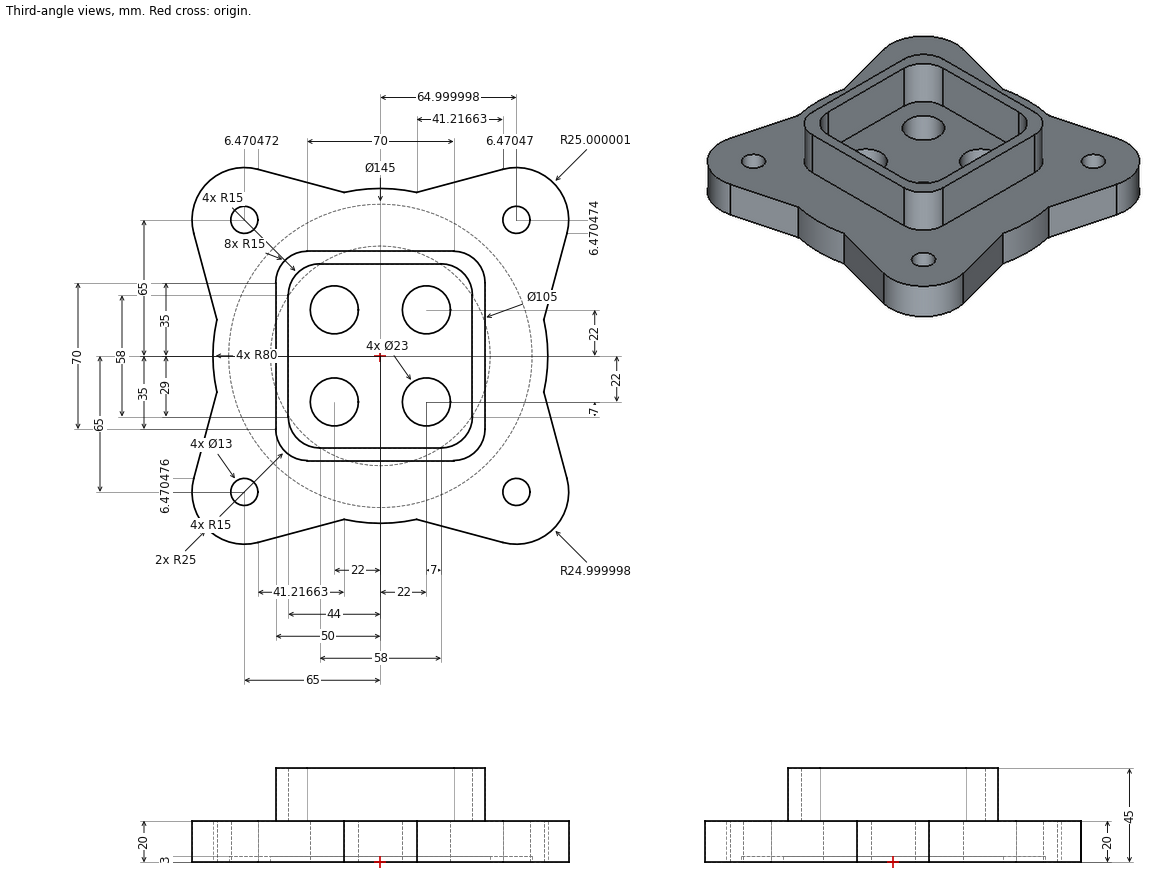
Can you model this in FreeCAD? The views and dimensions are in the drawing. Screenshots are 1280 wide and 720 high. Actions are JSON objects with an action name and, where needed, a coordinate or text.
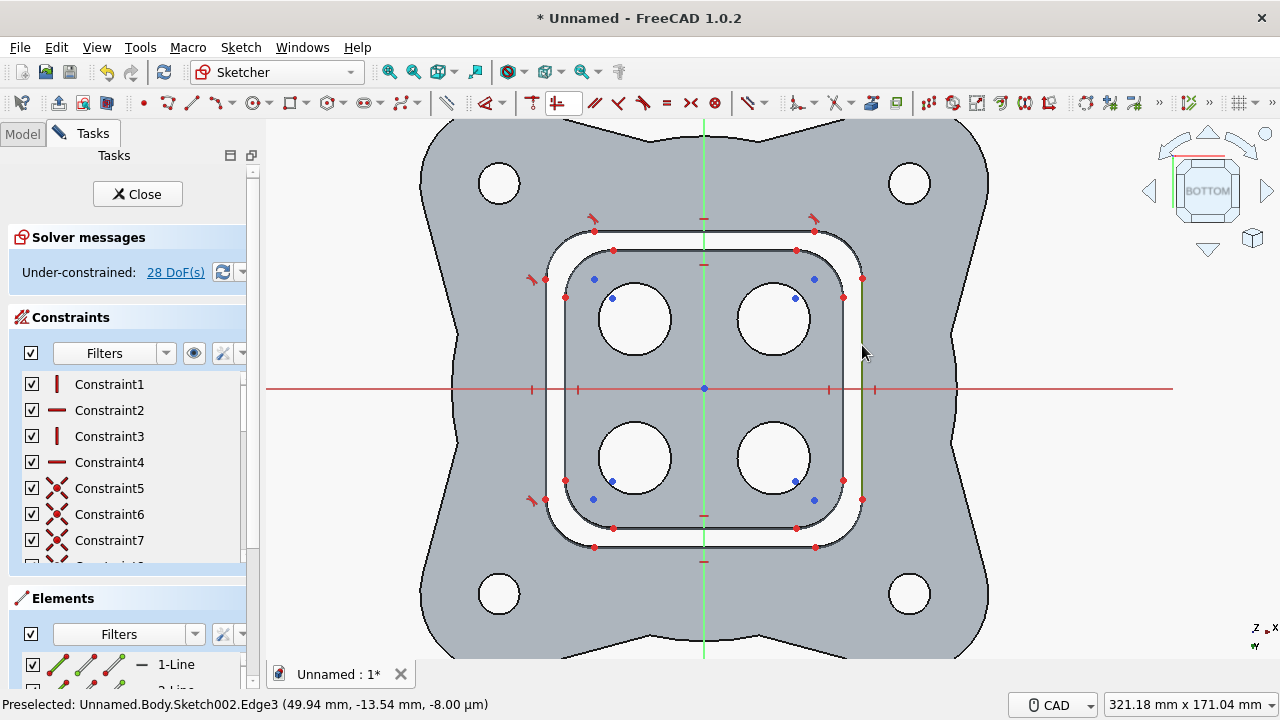
{"action": "left_click", "coordinate": [857, 258]}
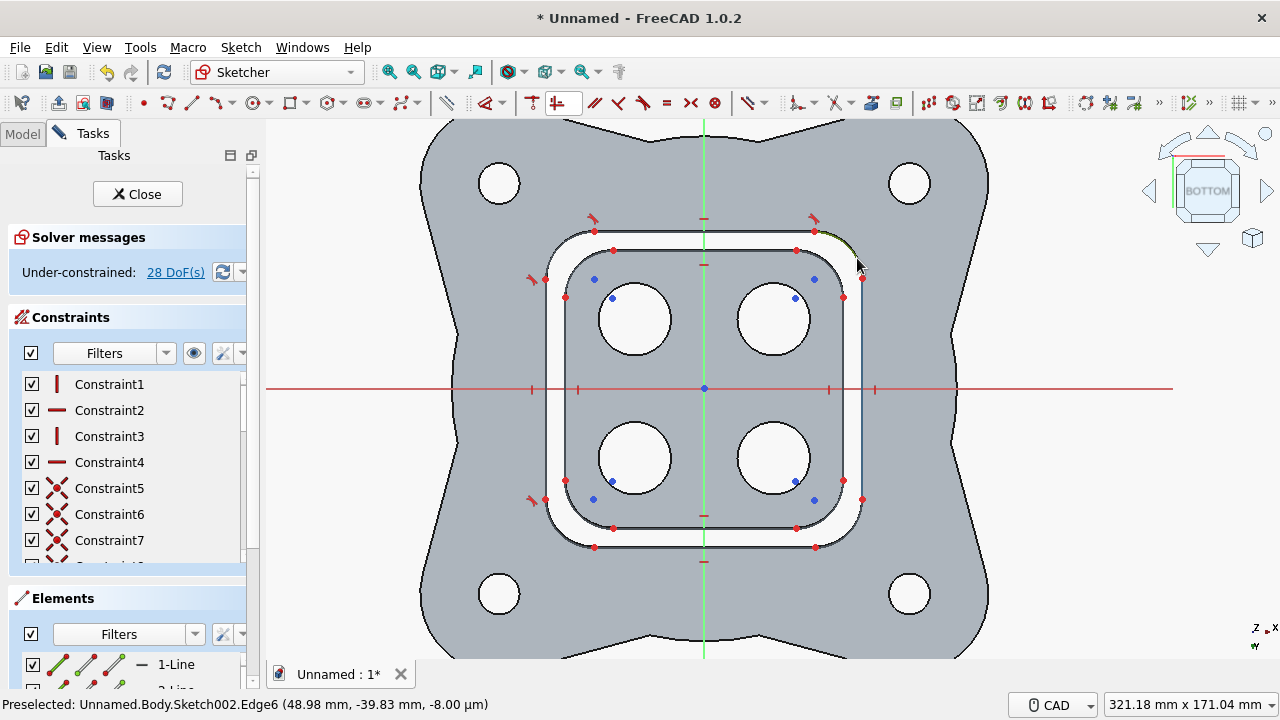
{"action": "left_click", "coordinate": [644, 104]}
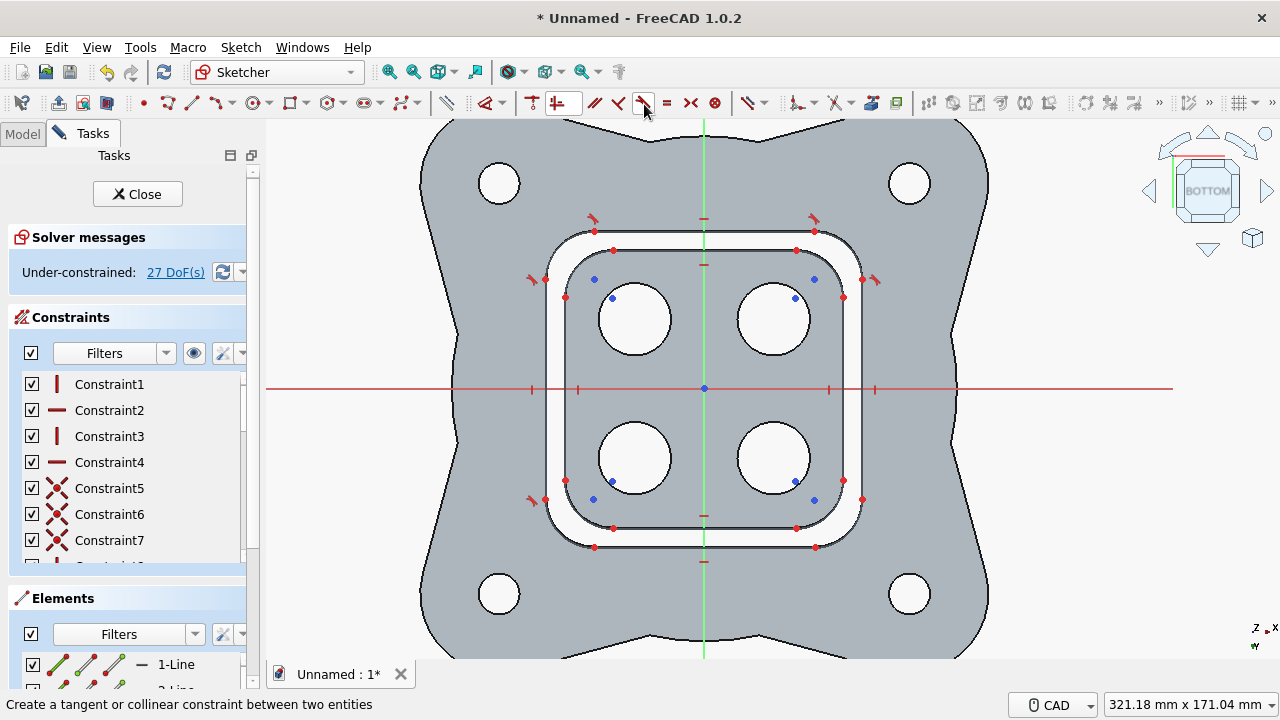
{"action": "left_click", "coordinate": [862, 346]}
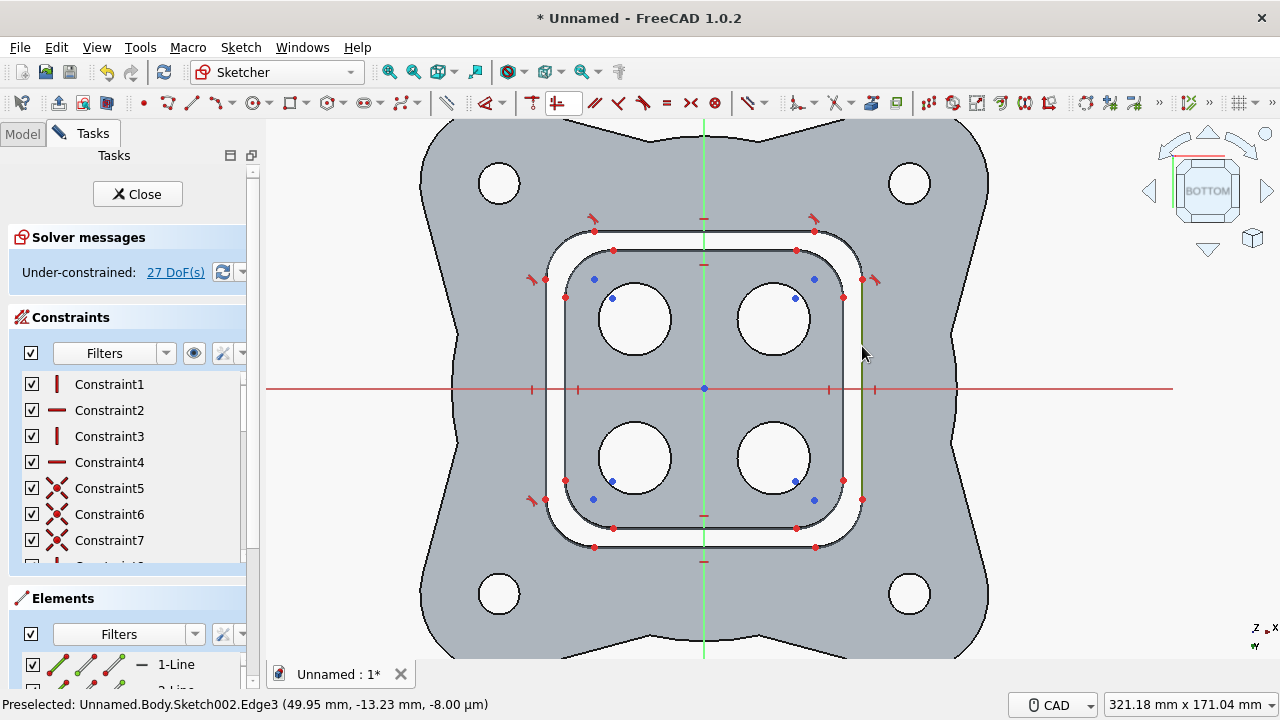
{"action": "left_click", "coordinate": [836, 543]}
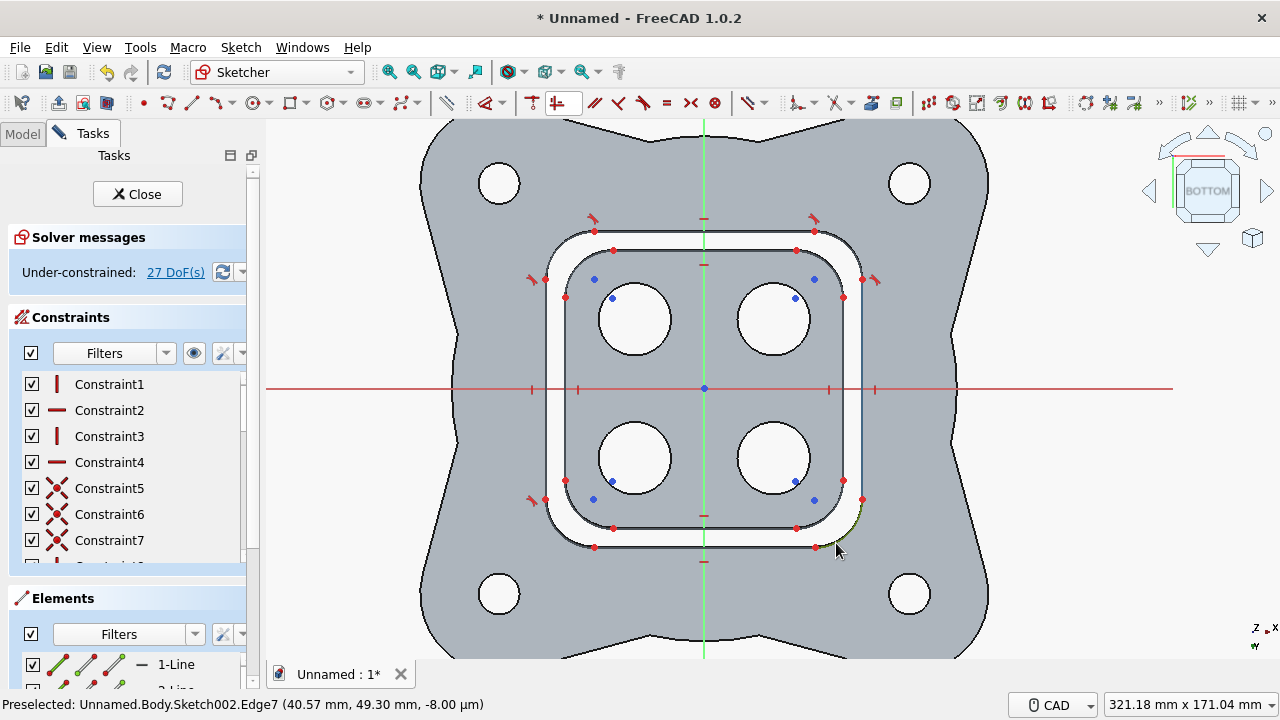
{"action": "left_click", "coordinate": [644, 104]}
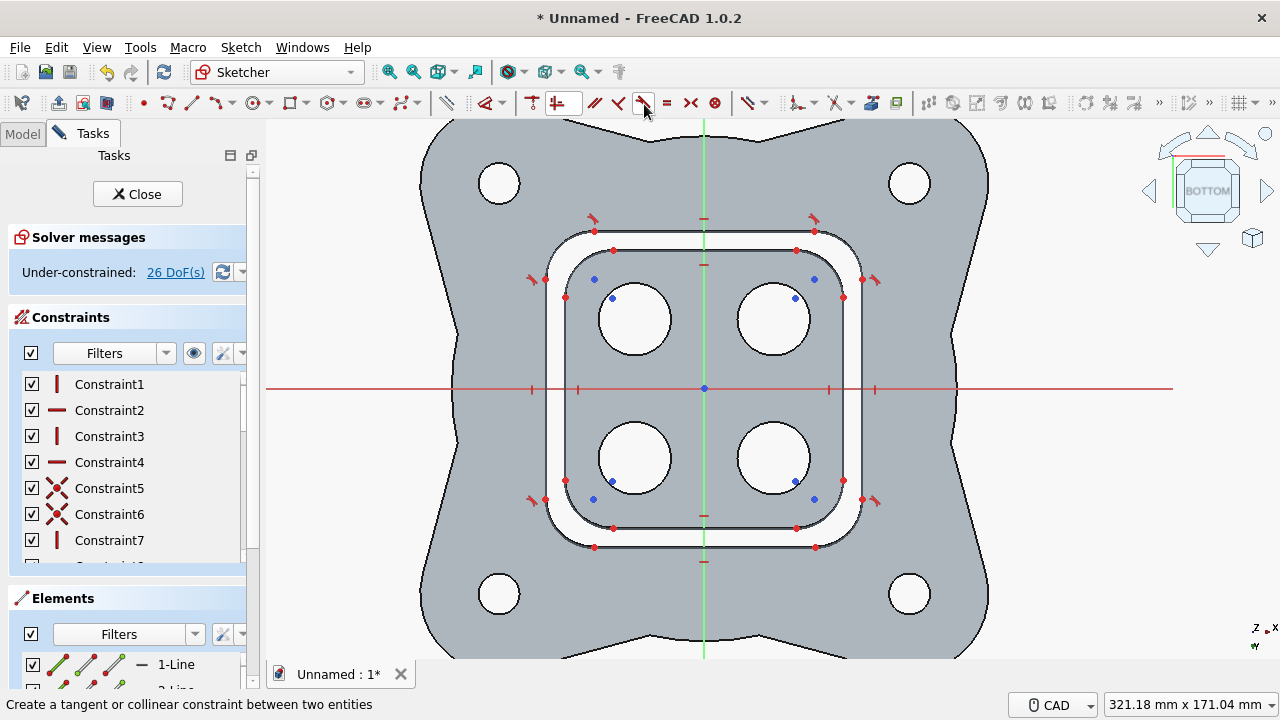
{"action": "left_click", "coordinate": [749, 548]}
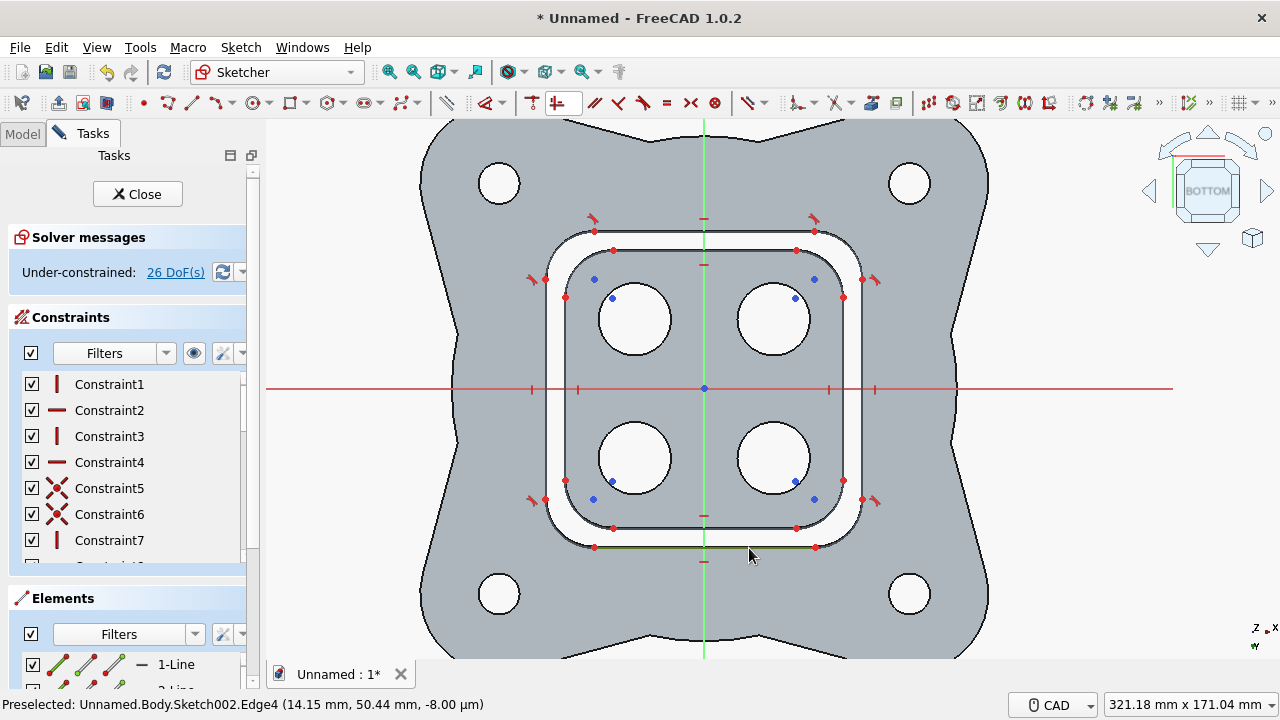
{"action": "left_click", "coordinate": [836, 543]}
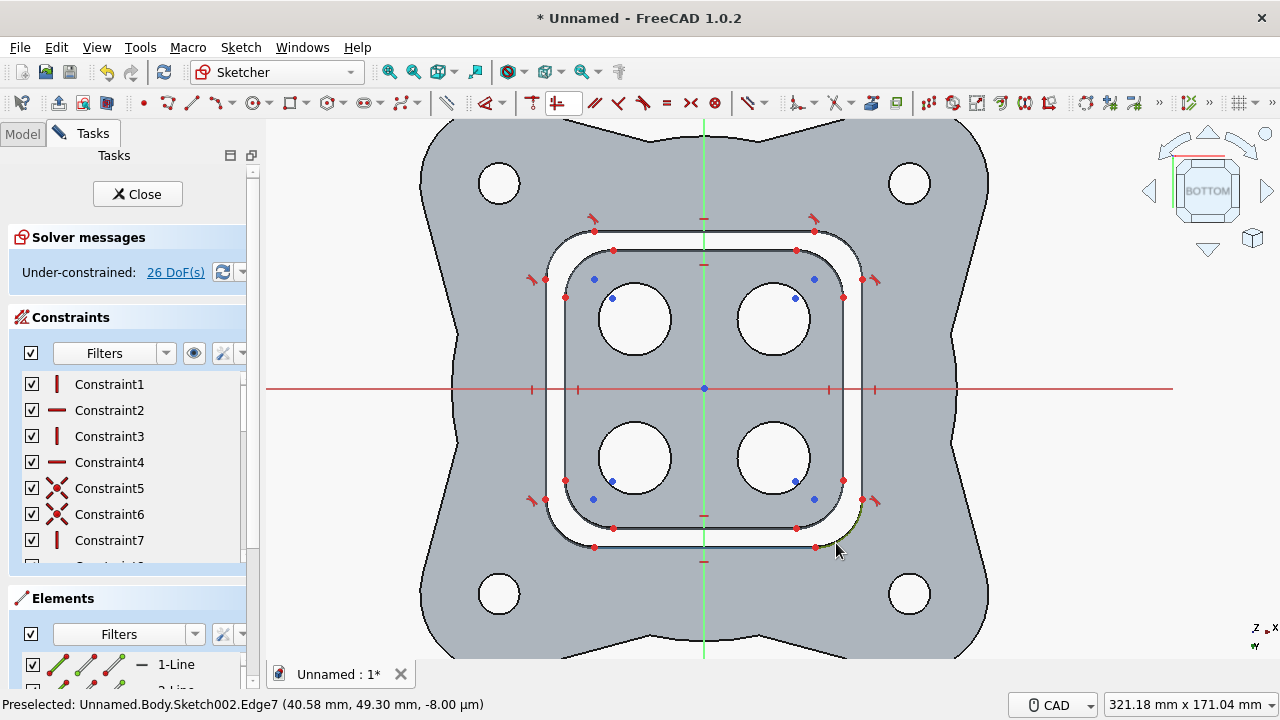
{"action": "left_click", "coordinate": [644, 104]}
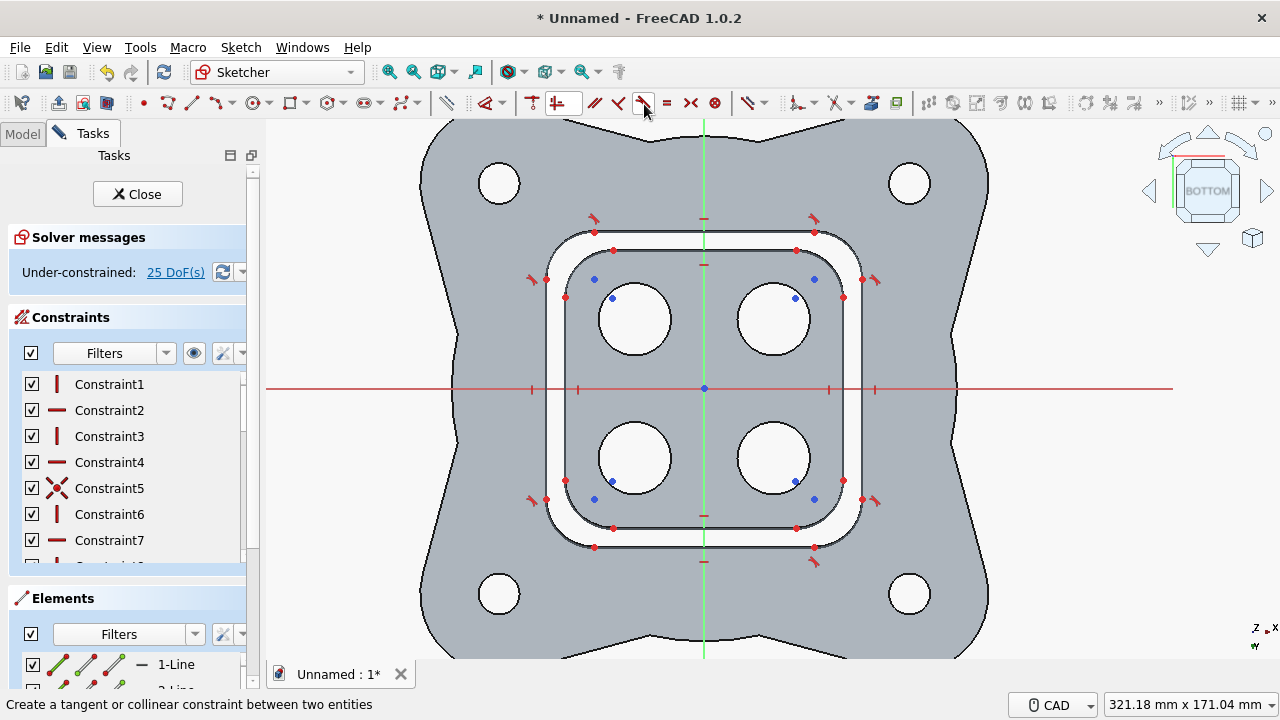
{"action": "left_click", "coordinate": [748, 548]}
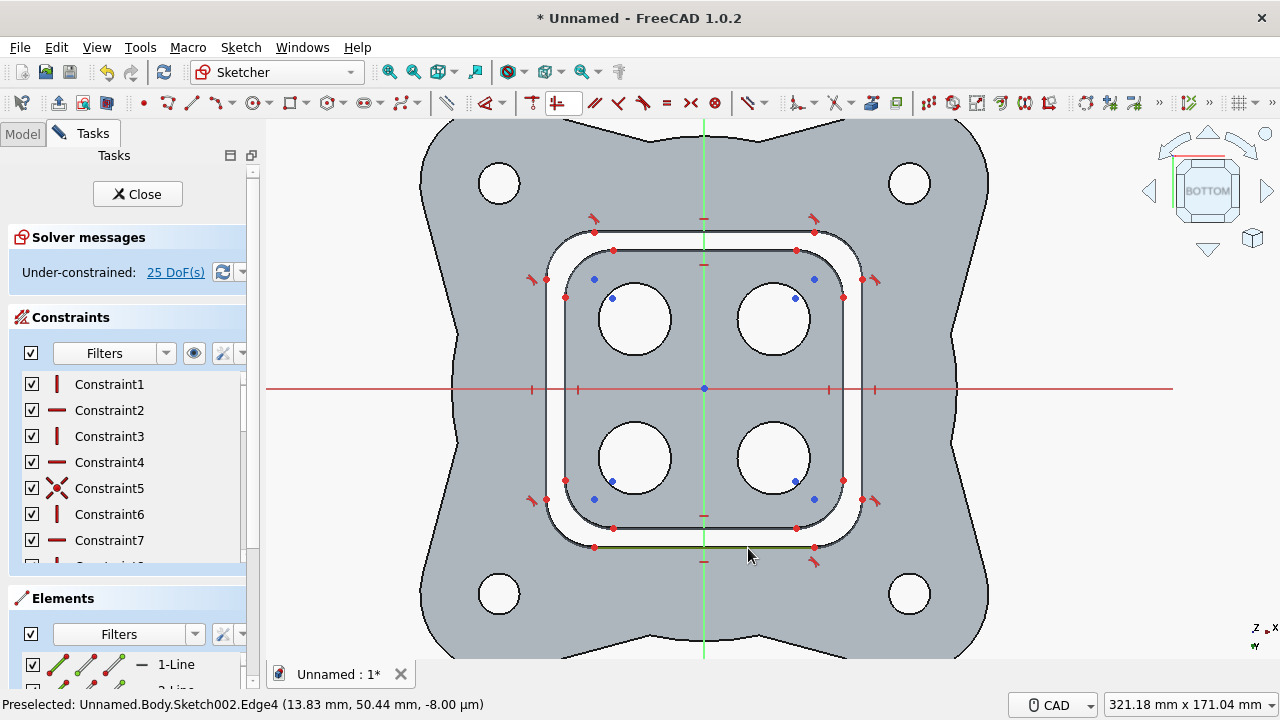
{"action": "left_click", "coordinate": [551, 522]}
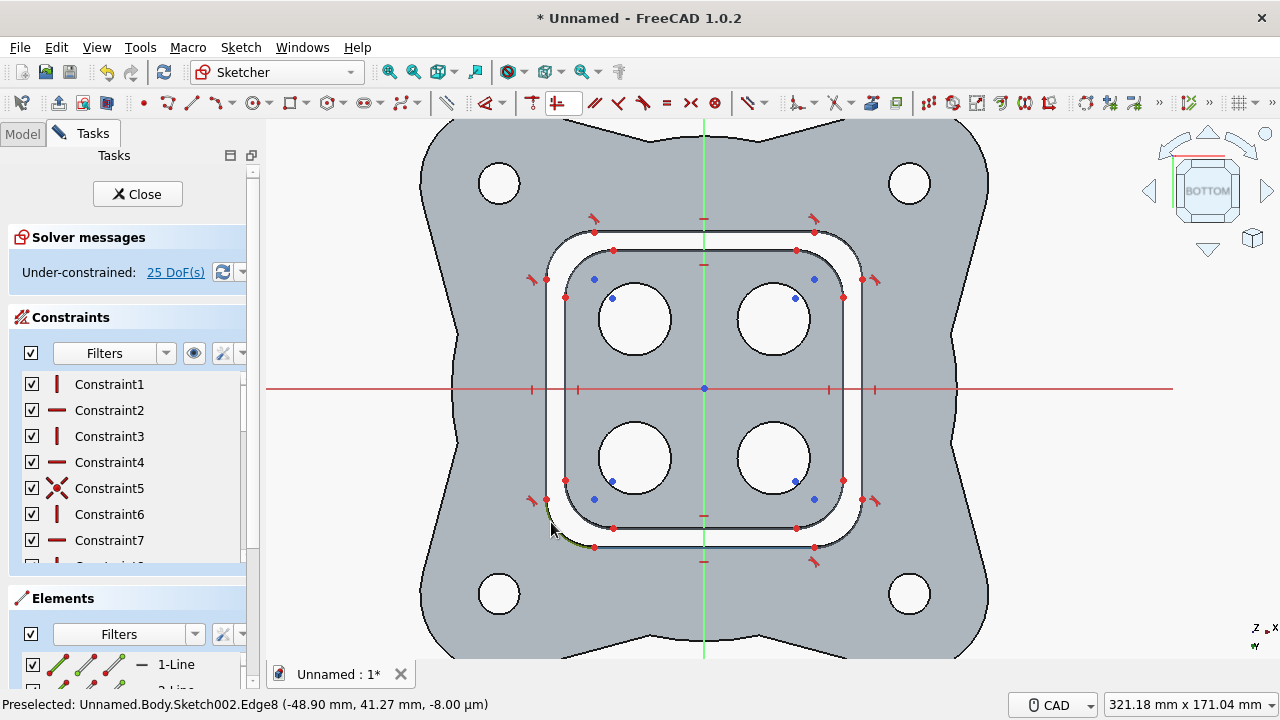
{"action": "key", "text": "t"}